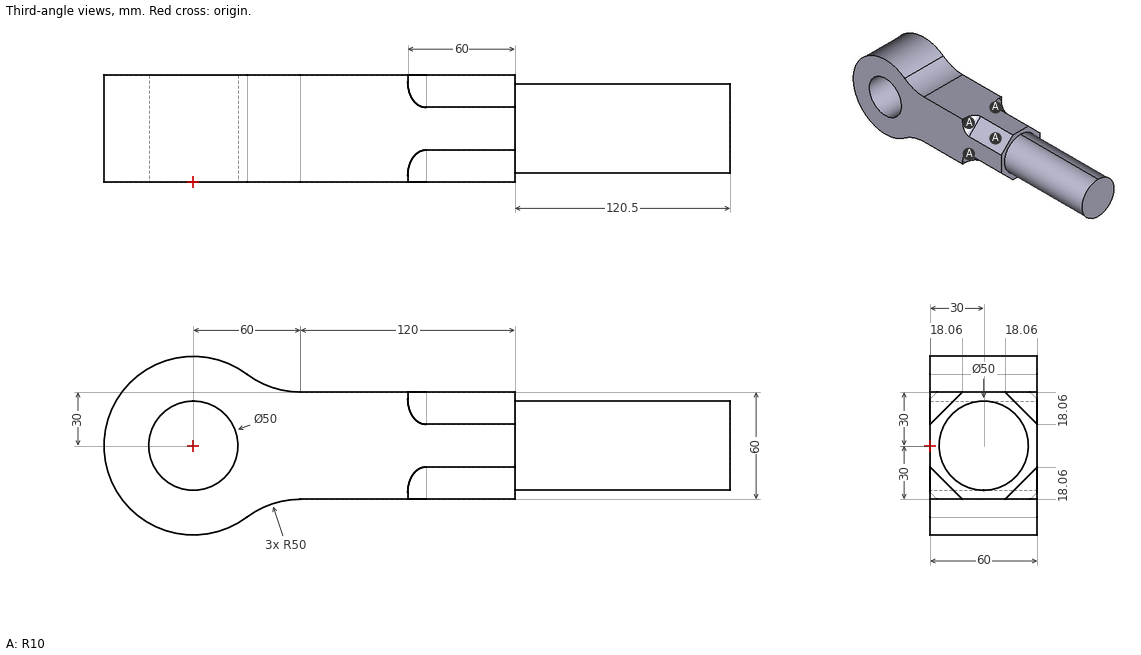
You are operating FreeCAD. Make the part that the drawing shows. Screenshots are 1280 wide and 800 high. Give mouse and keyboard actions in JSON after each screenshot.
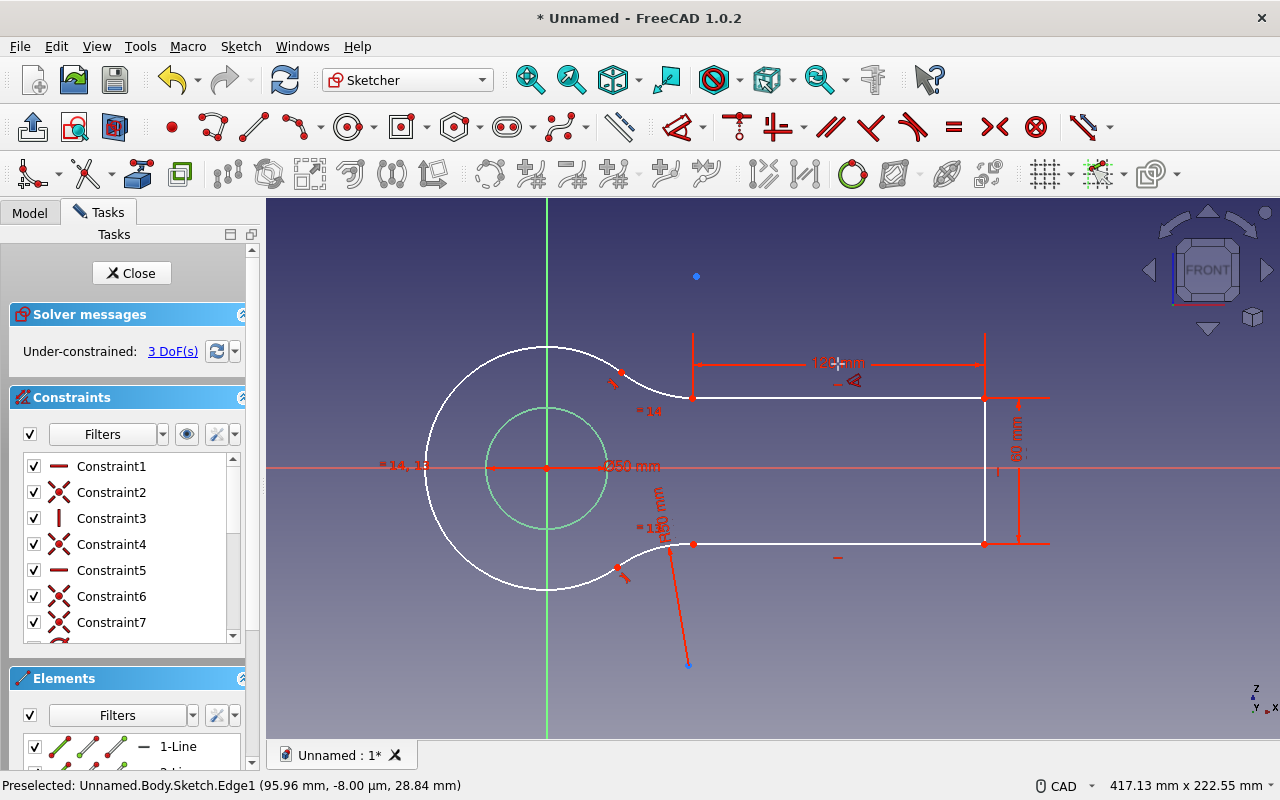
{"action": "left_click", "coordinate": [897, 544]}
{"action": "left_click", "coordinate": [839, 578]}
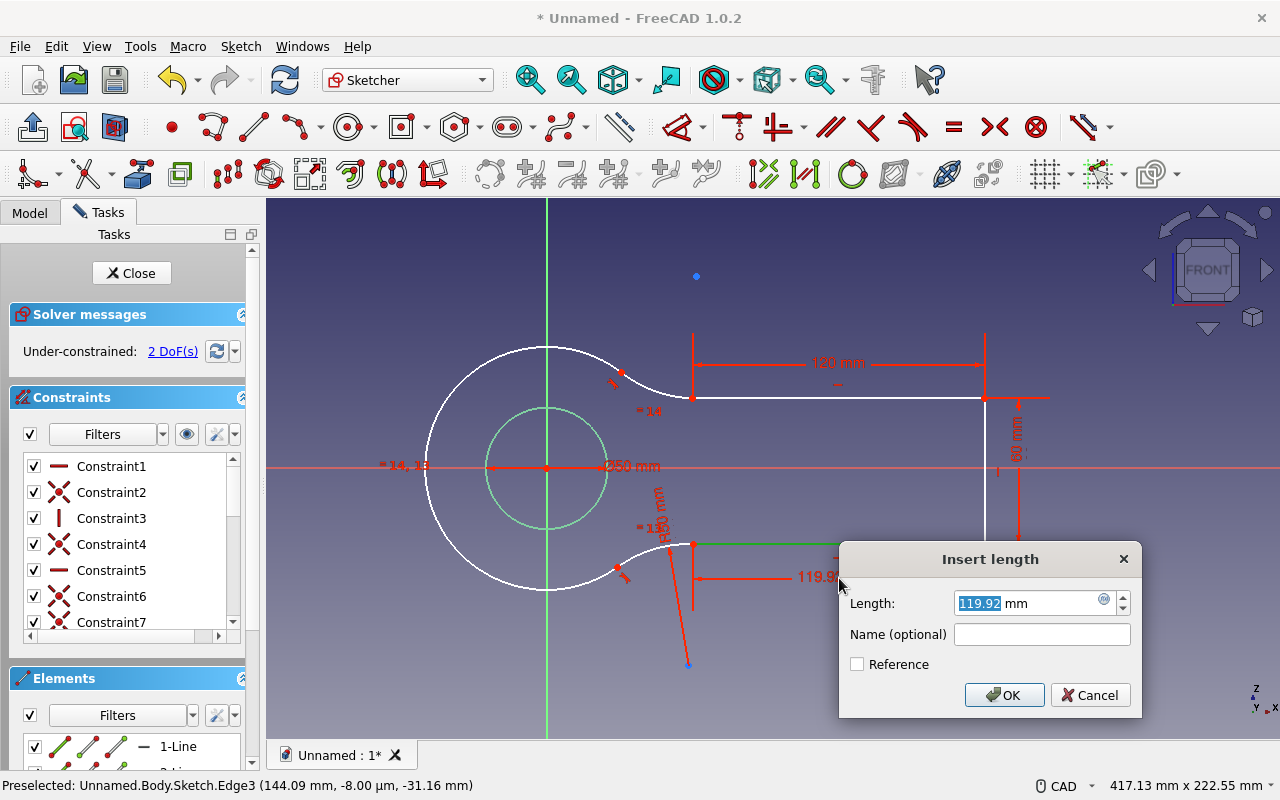
{"action": "type", "text": "120"}
{"action": "key", "text": "Return"}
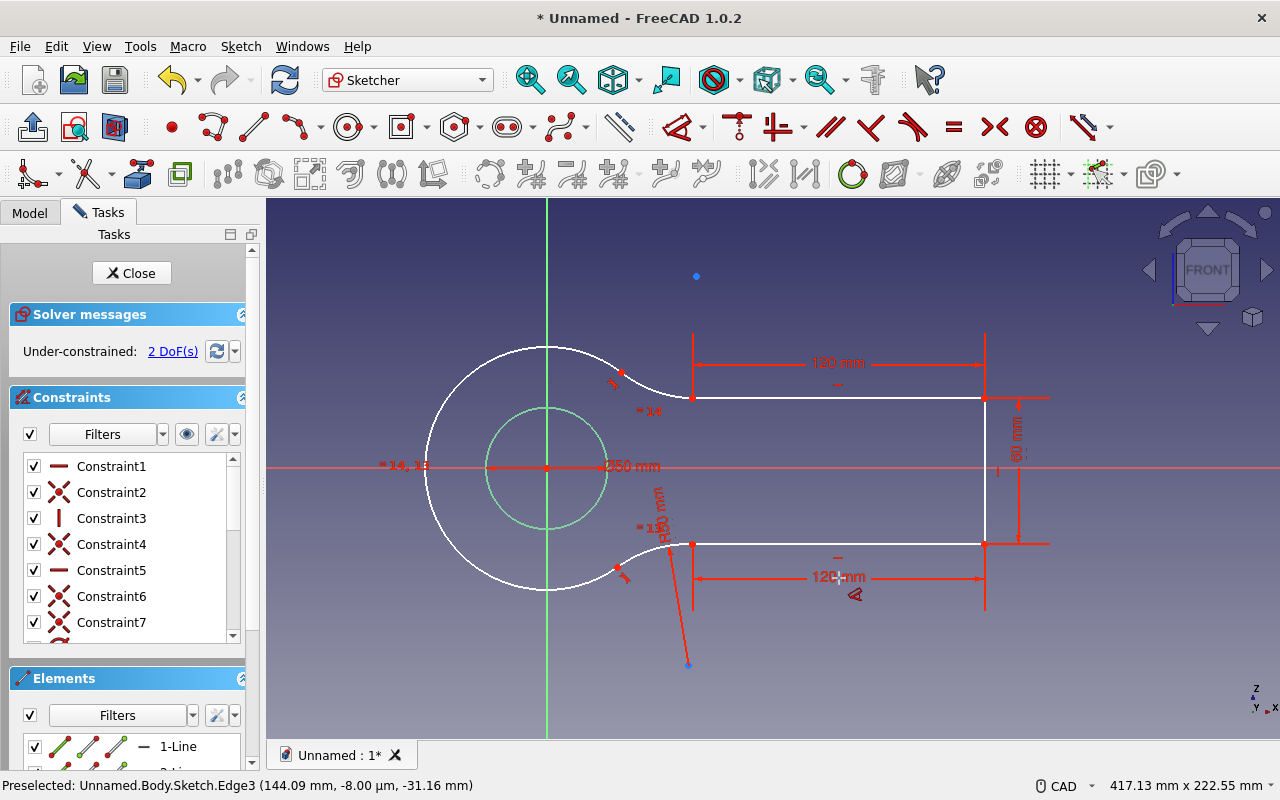
{"action": "left_click", "coordinate": [693, 398]}
{"action": "left_click", "coordinate": [653, 364]}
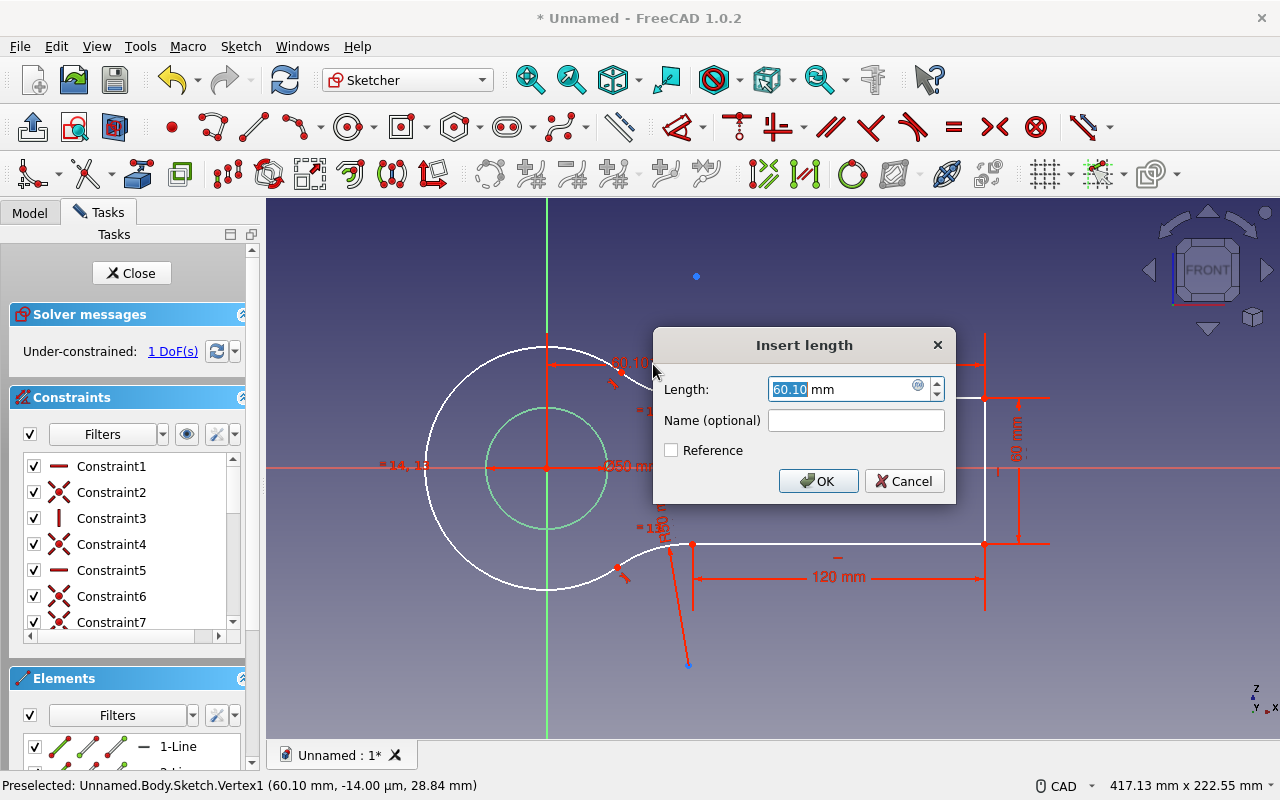
{"action": "type", "text": "60"}
{"action": "key", "text": "Return"}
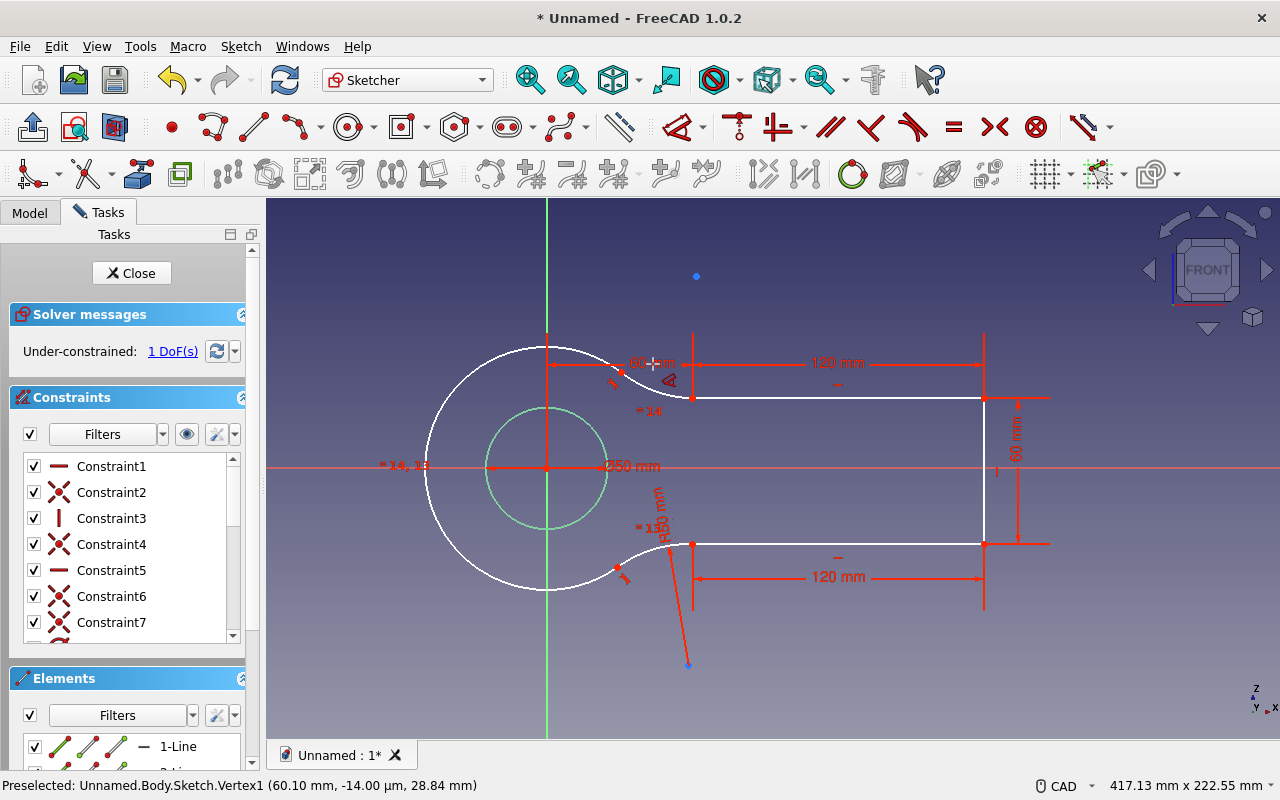
{"action": "left_click", "coordinate": [693, 398]}
{"action": "left_click", "coordinate": [513, 449]}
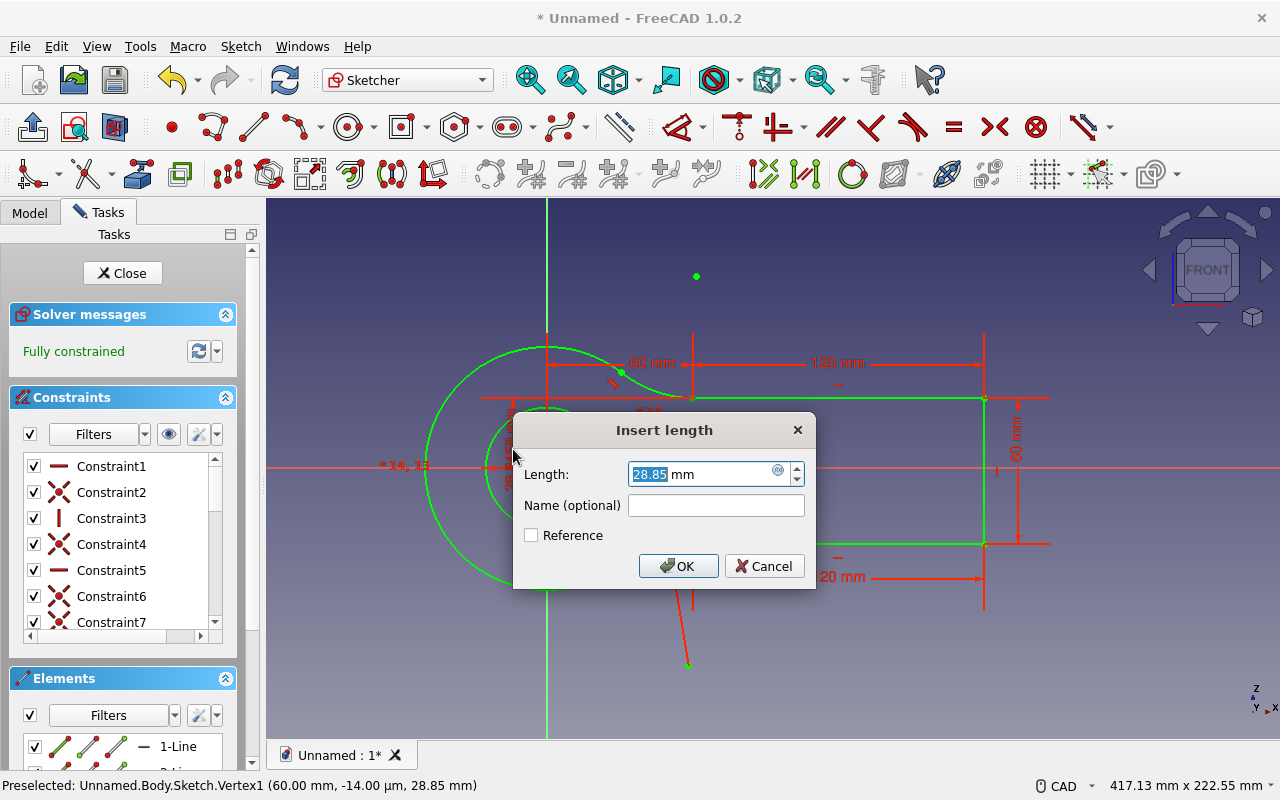
{"action": "type", "text": "30"}
{"action": "key", "text": "Return"}
{"action": "key", "text": "Escape"}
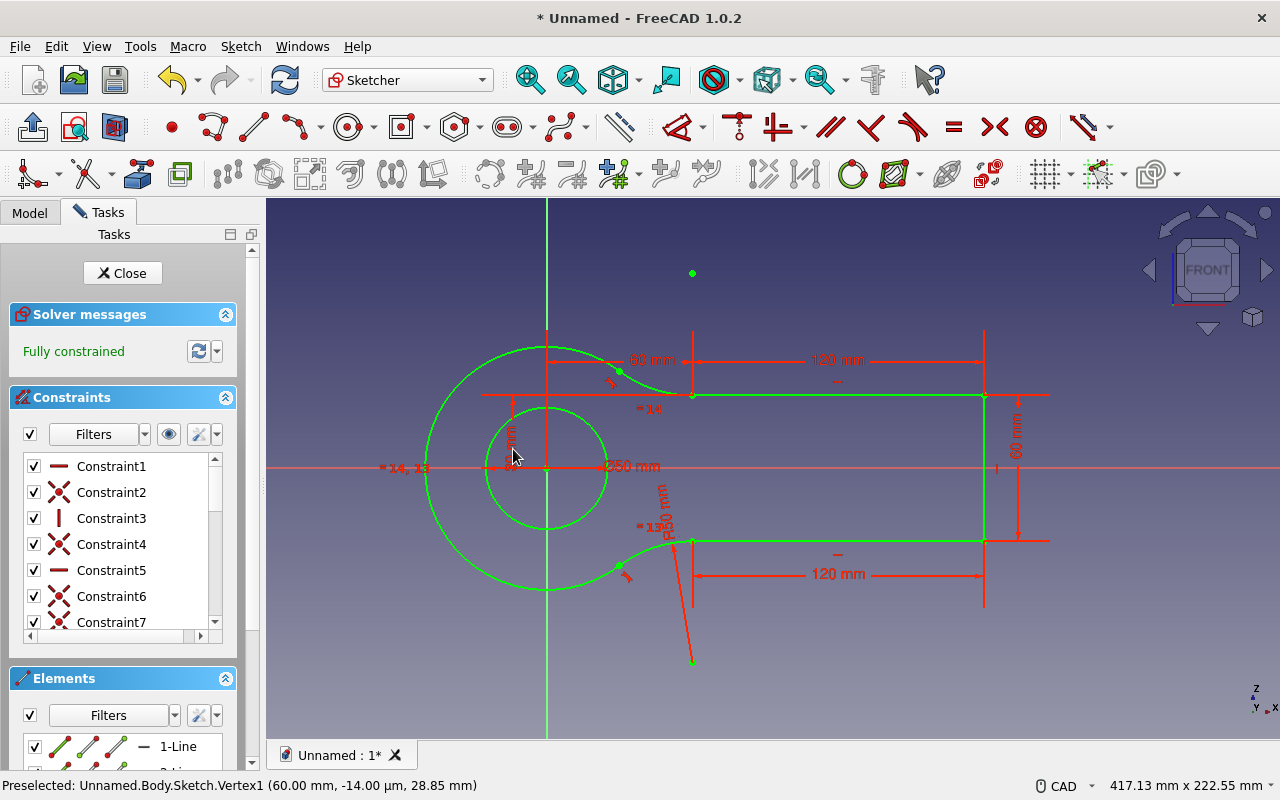
{"action": "left_click", "coordinate": [123, 273]}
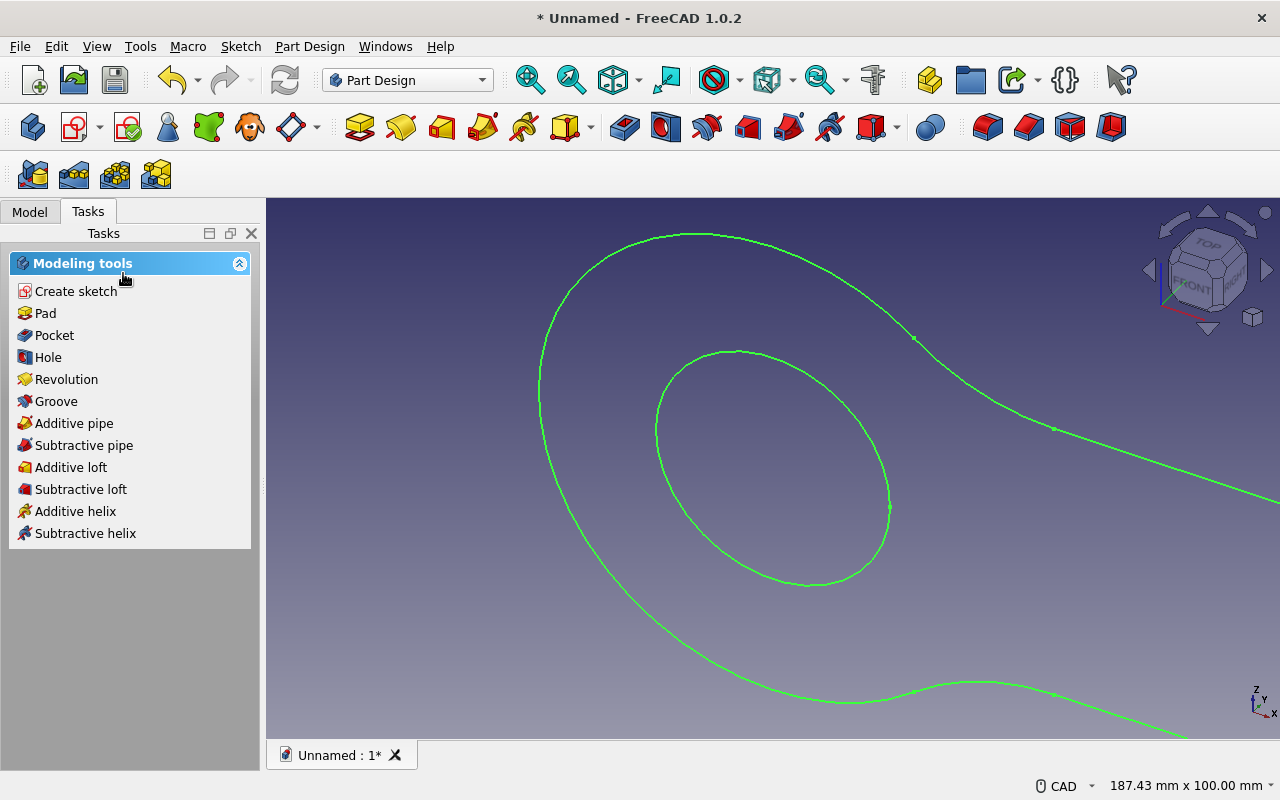
{"action": "left_click", "coordinate": [360, 128]}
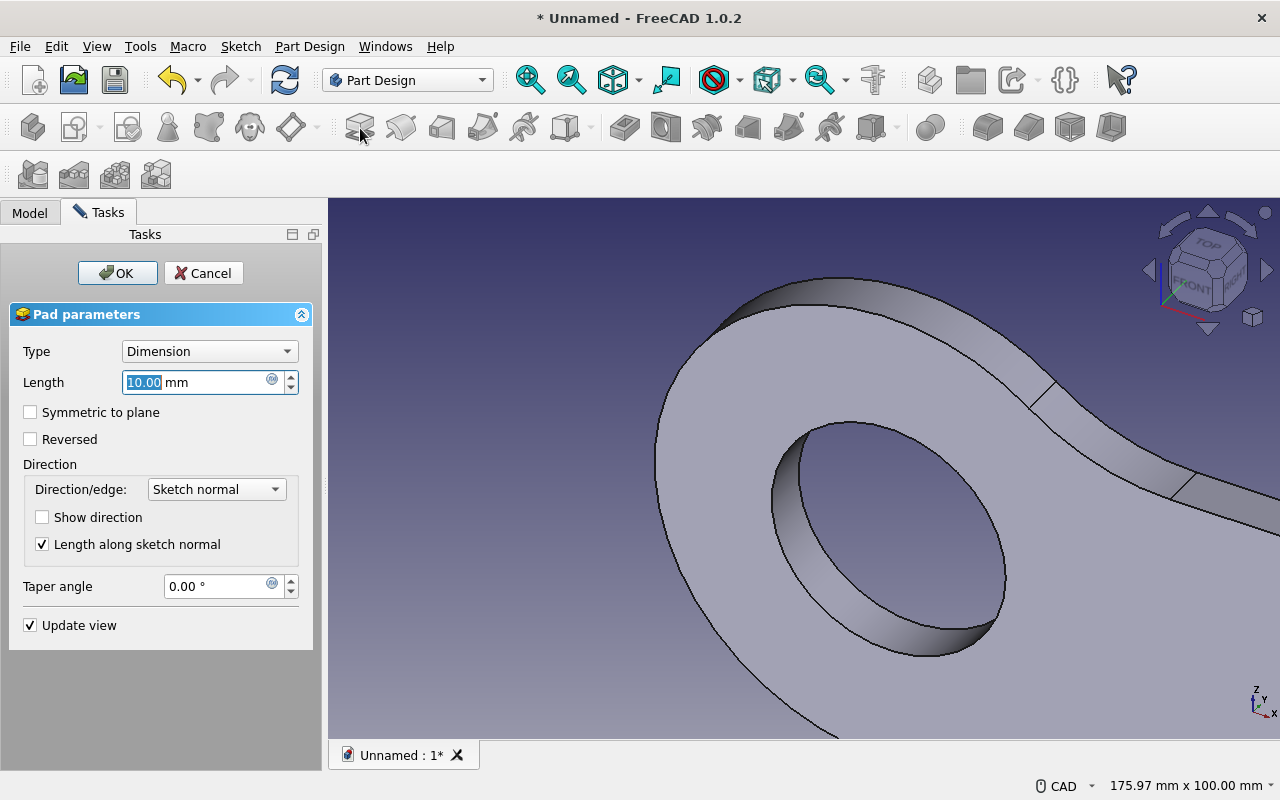
{"action": "type", "text": "60"}
{"action": "key", "text": "Tab"}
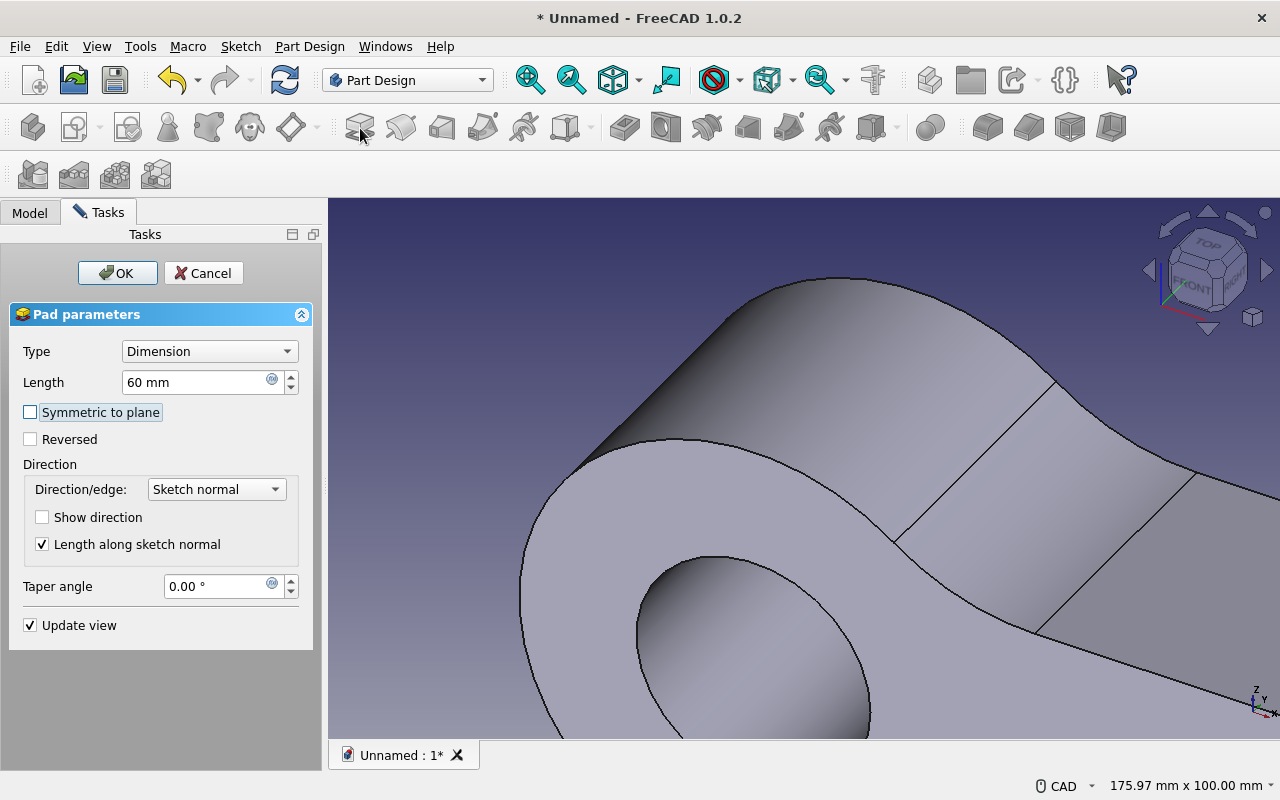
{"action": "left_click", "coordinate": [31, 439]}